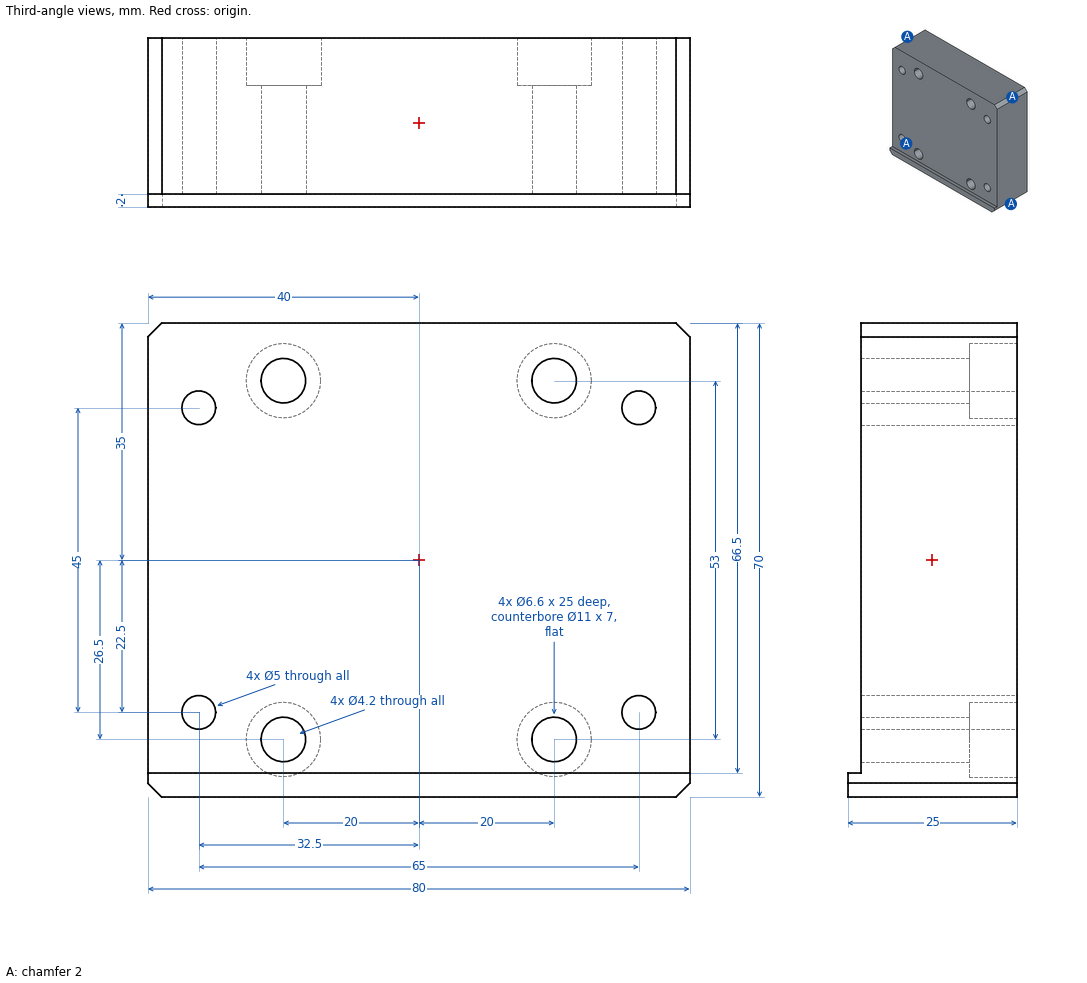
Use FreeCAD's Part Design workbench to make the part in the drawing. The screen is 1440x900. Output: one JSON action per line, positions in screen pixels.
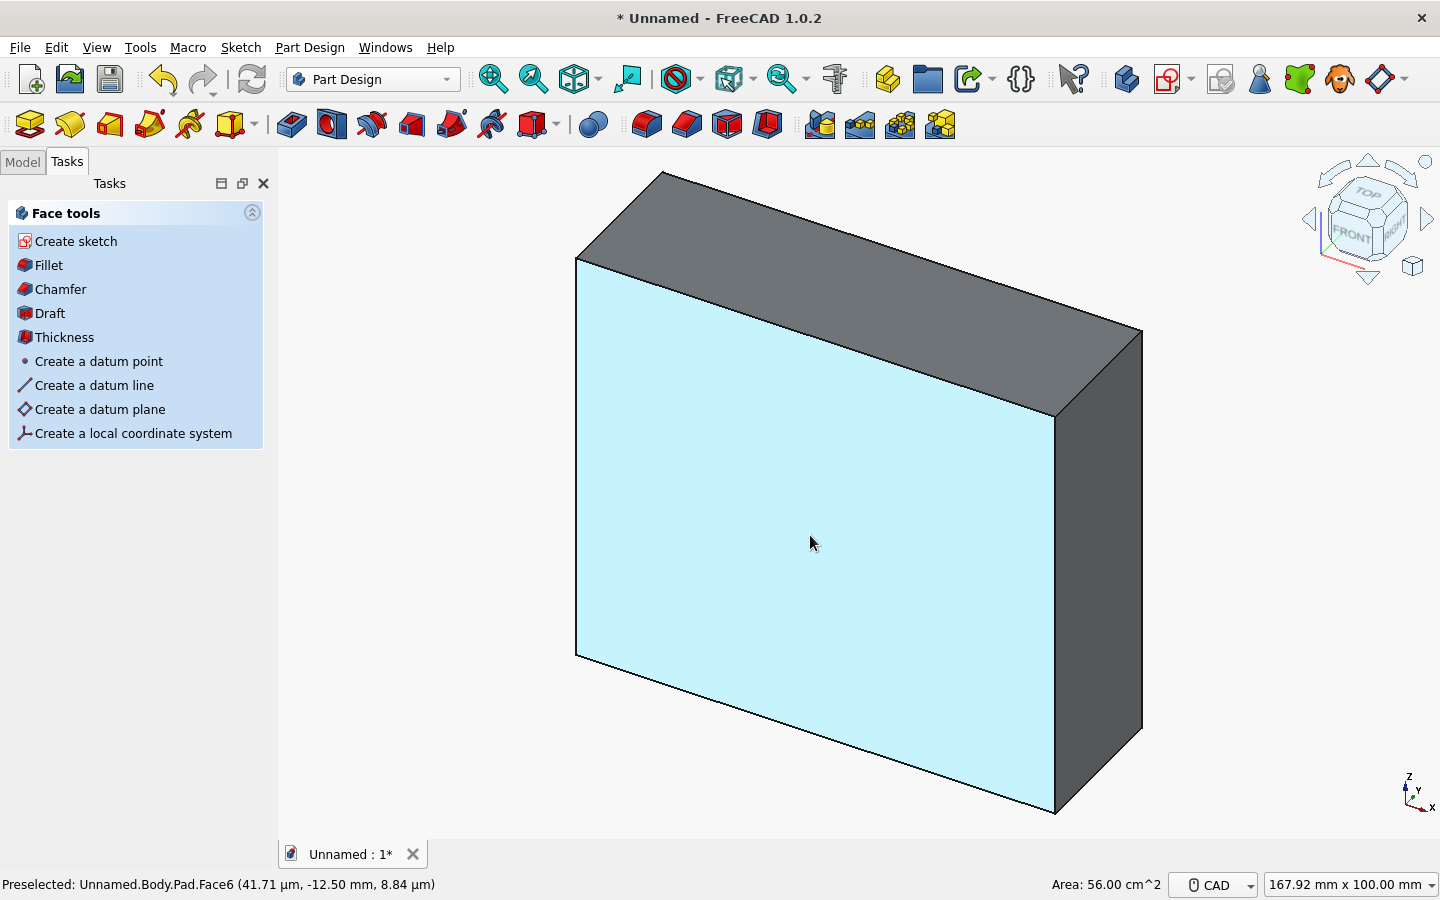
{"action": "left_click", "coordinate": [1168, 80]}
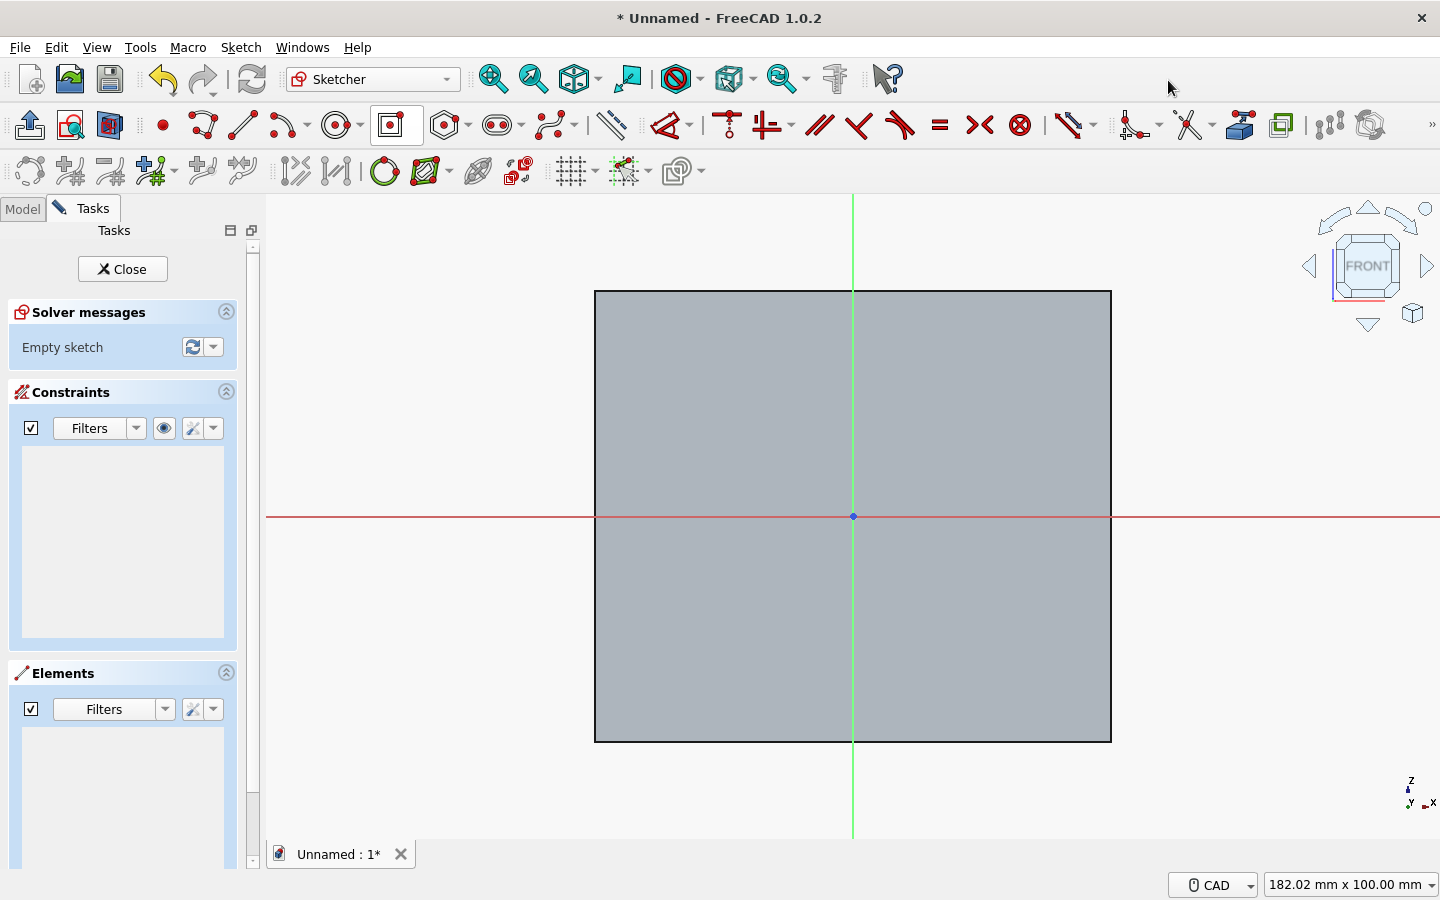
{"action": "key", "text": "g r"}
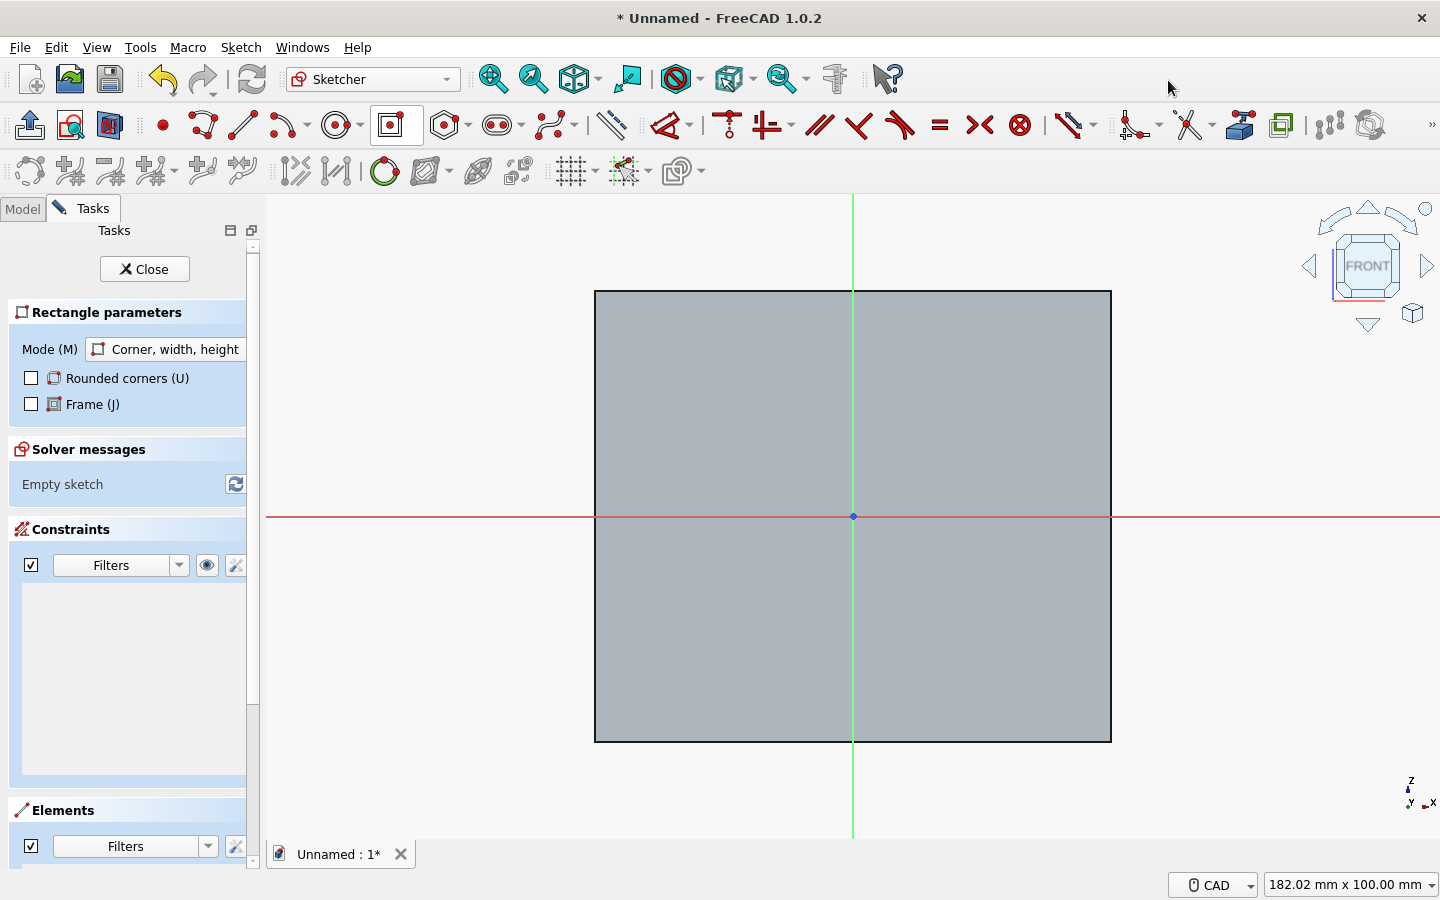
{"action": "left_click", "coordinate": [595, 291]}
{"action": "mouse_move", "coordinate": [1111, 720]}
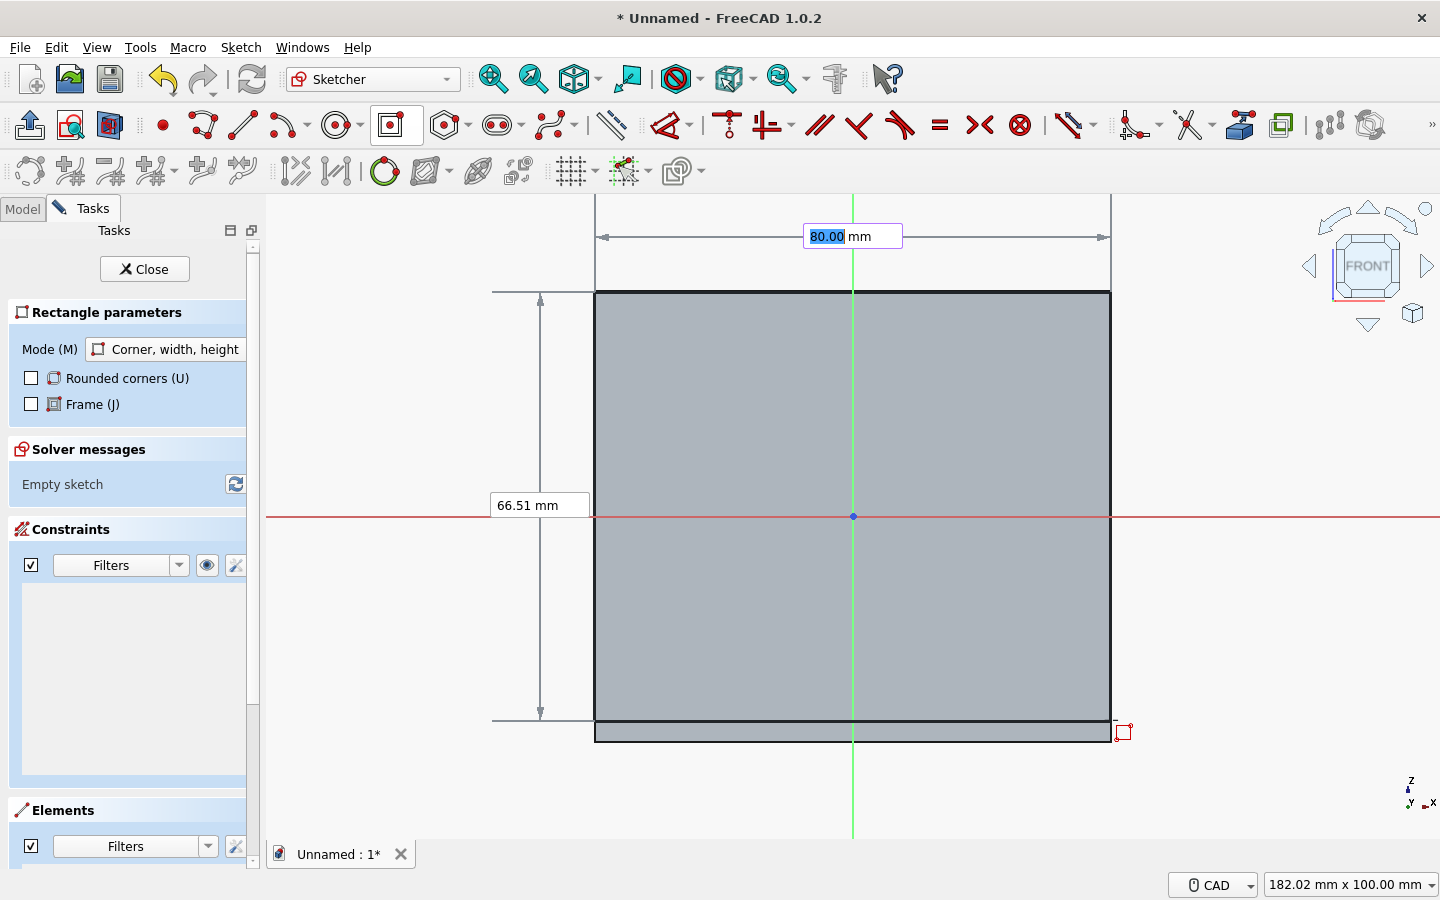
{"action": "type", "text": "80"}
{"action": "key", "text": "Tab"}
{"action": "type", "text": "66.5"}
{"action": "key", "text": "Return"}
{"action": "key", "text": "Escape"}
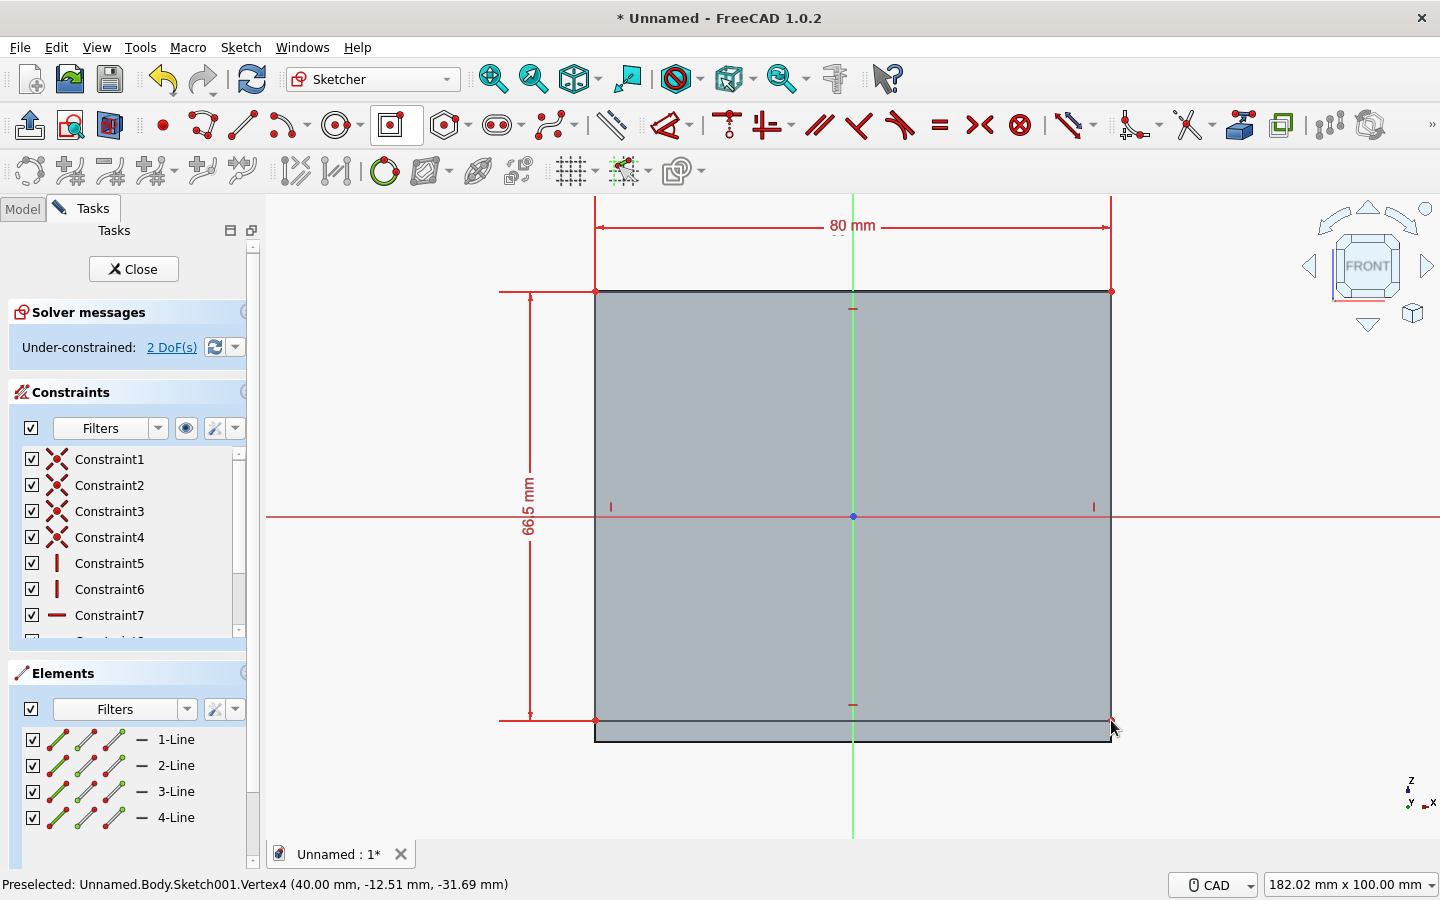
{"action": "left_click", "coordinate": [595, 292]}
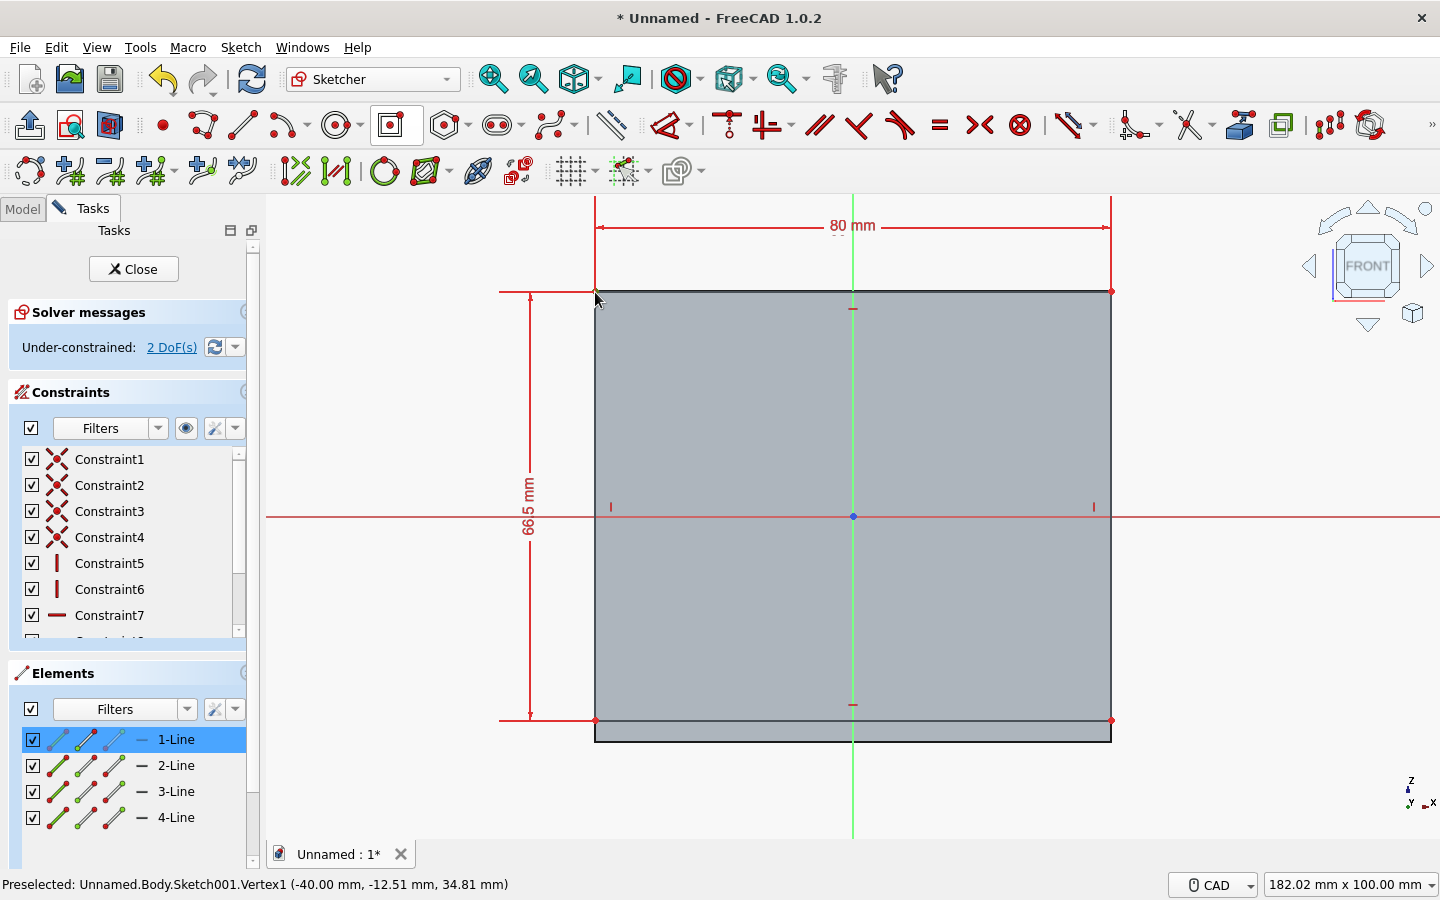
{"action": "key", "text": "l"}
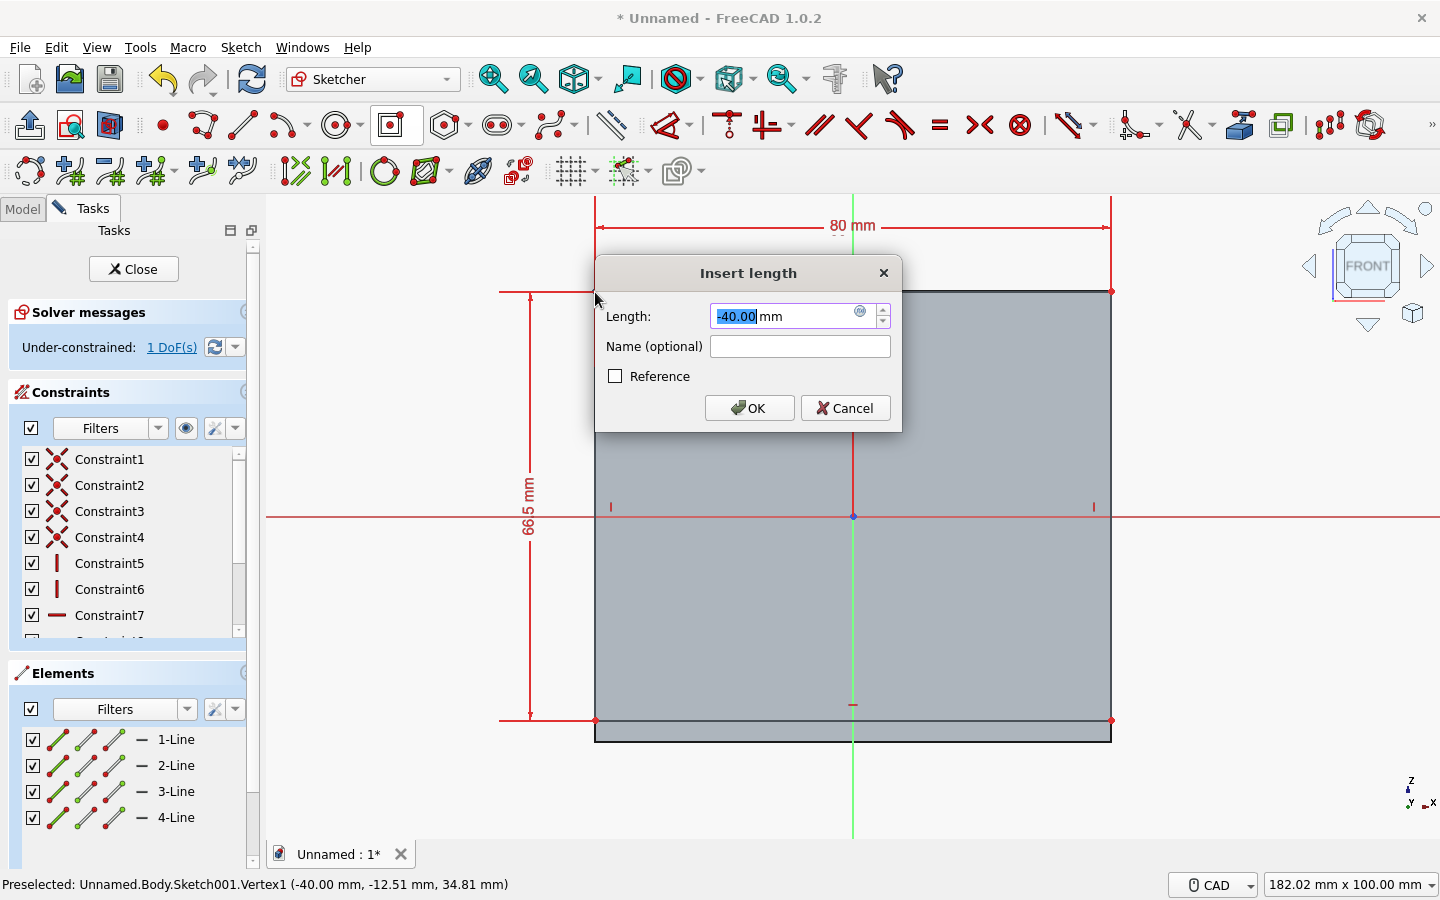
{"action": "type", "text": "-40"}
{"action": "key", "text": "Return"}